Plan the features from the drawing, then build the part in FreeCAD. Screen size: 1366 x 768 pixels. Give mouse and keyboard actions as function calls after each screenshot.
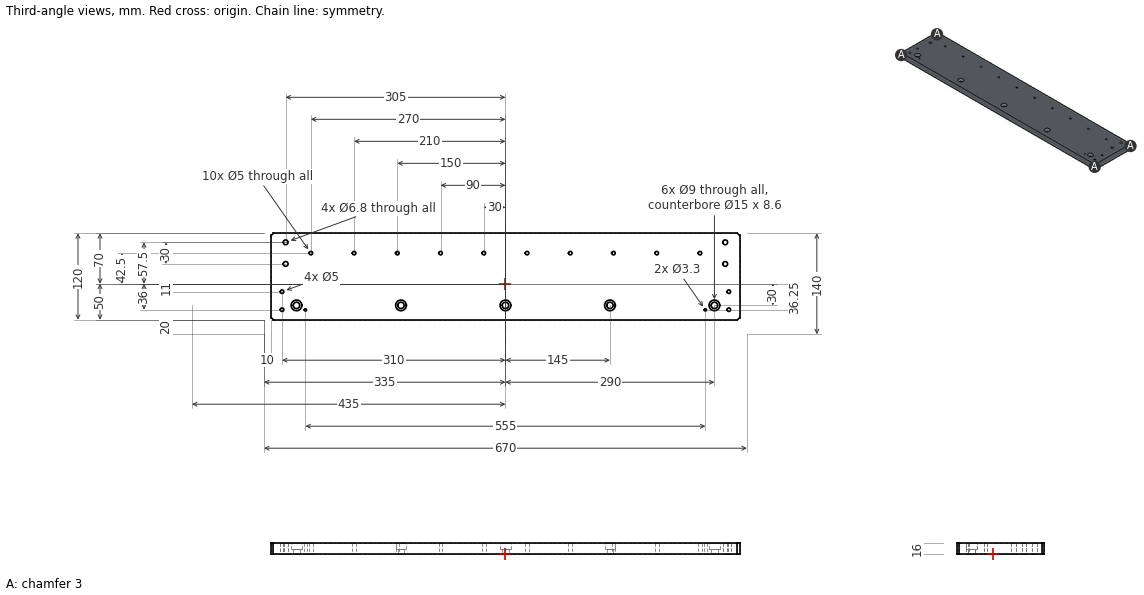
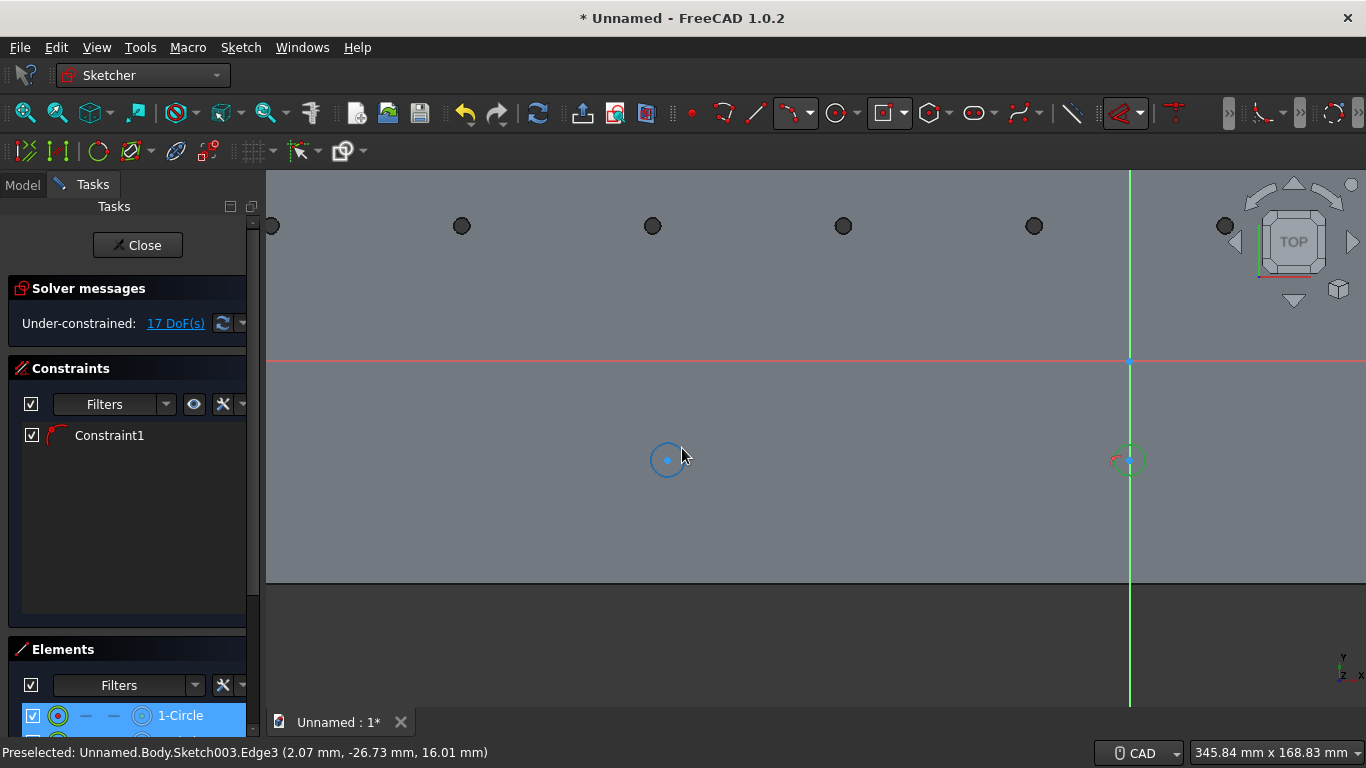
click(680, 448)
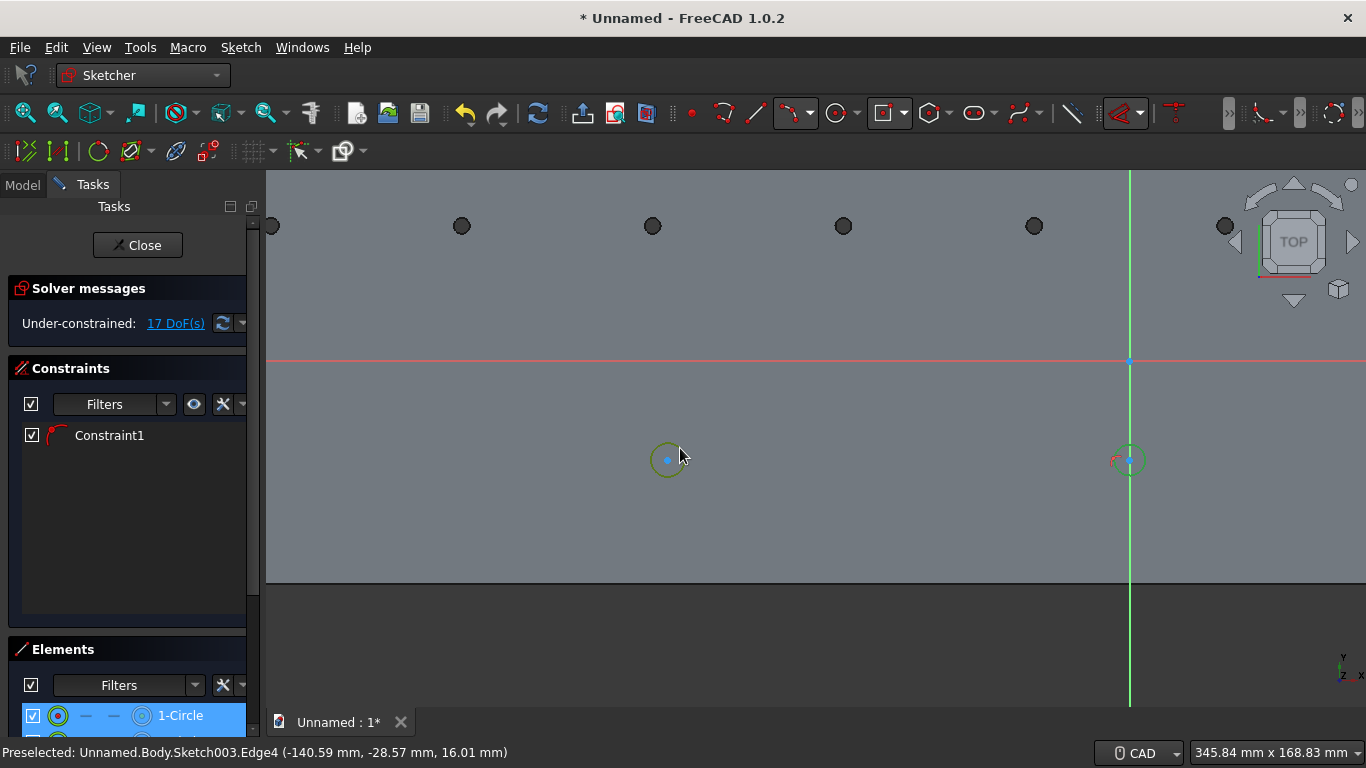
scroll(682, 448, down, 6)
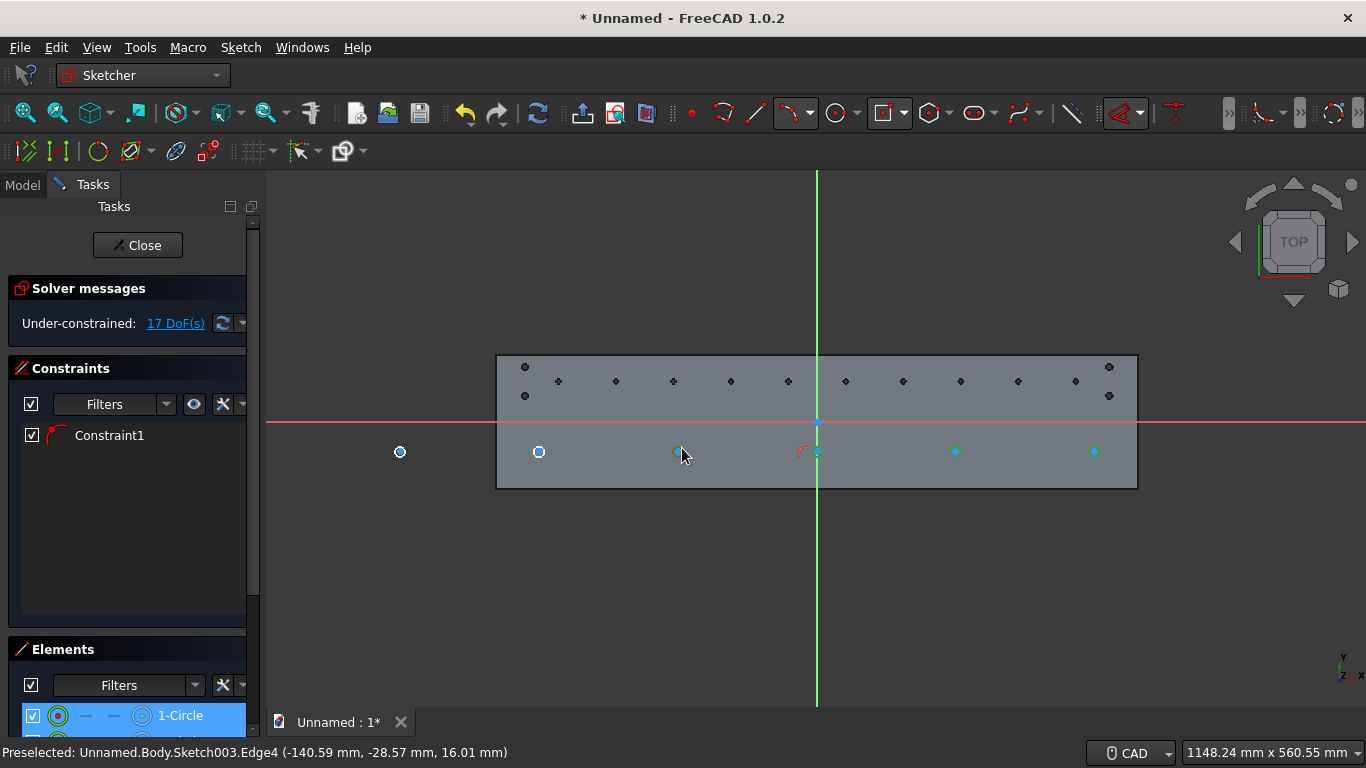
scroll(543, 448, up, 5)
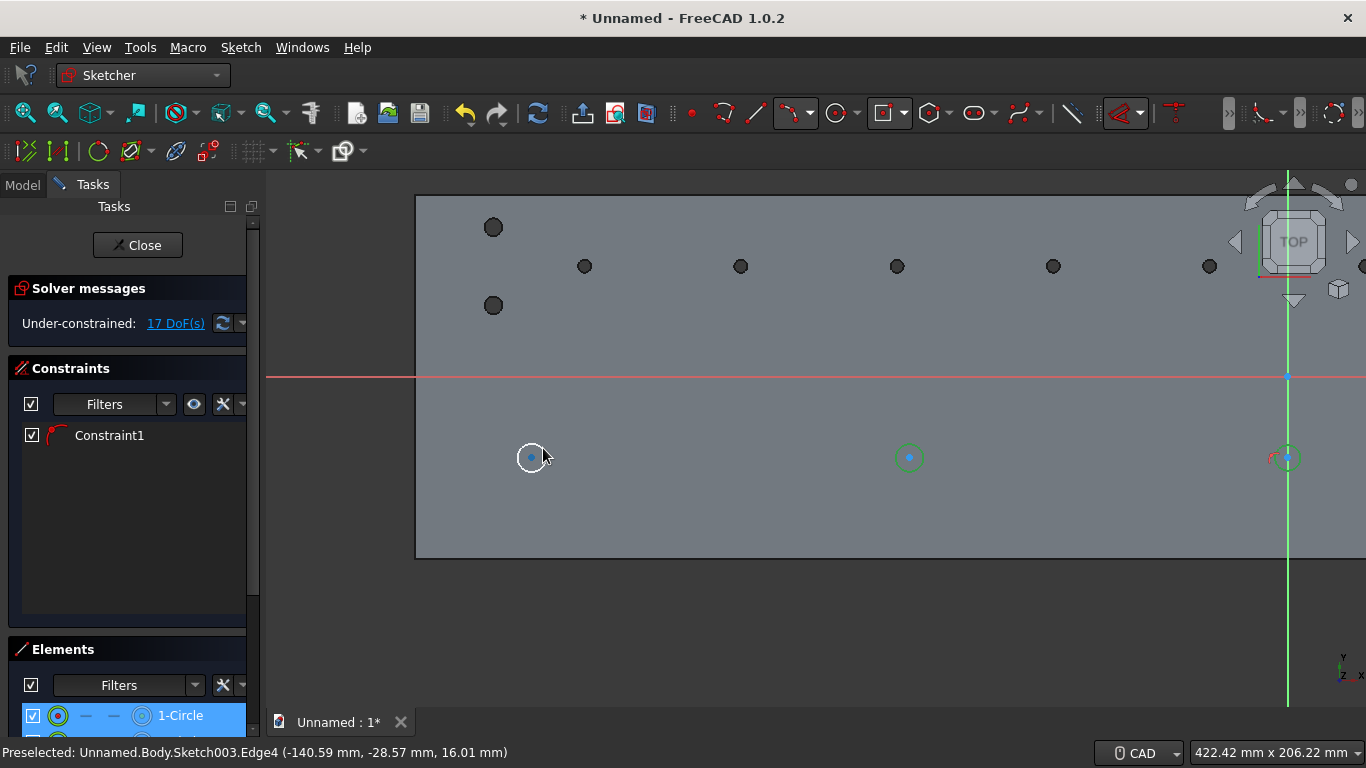
click(542, 448)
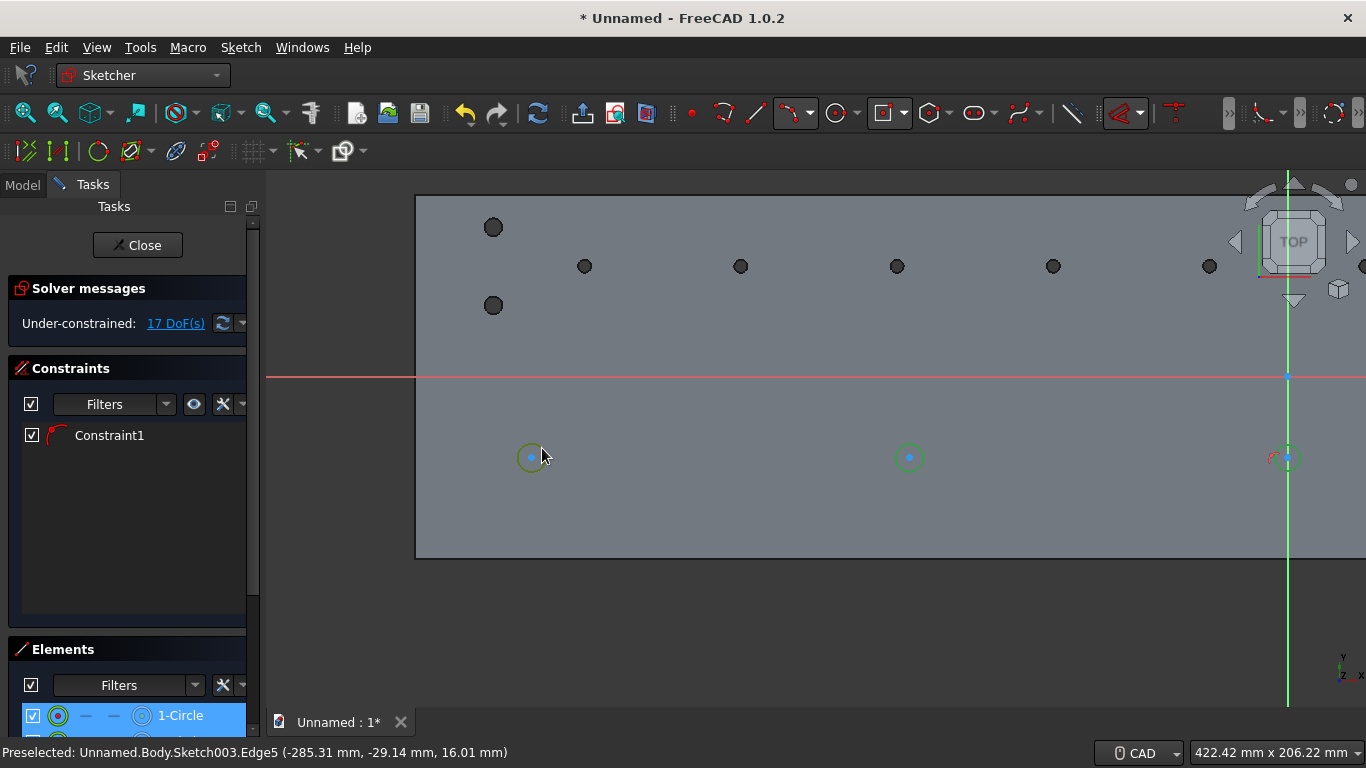
scroll(543, 448, down, 5)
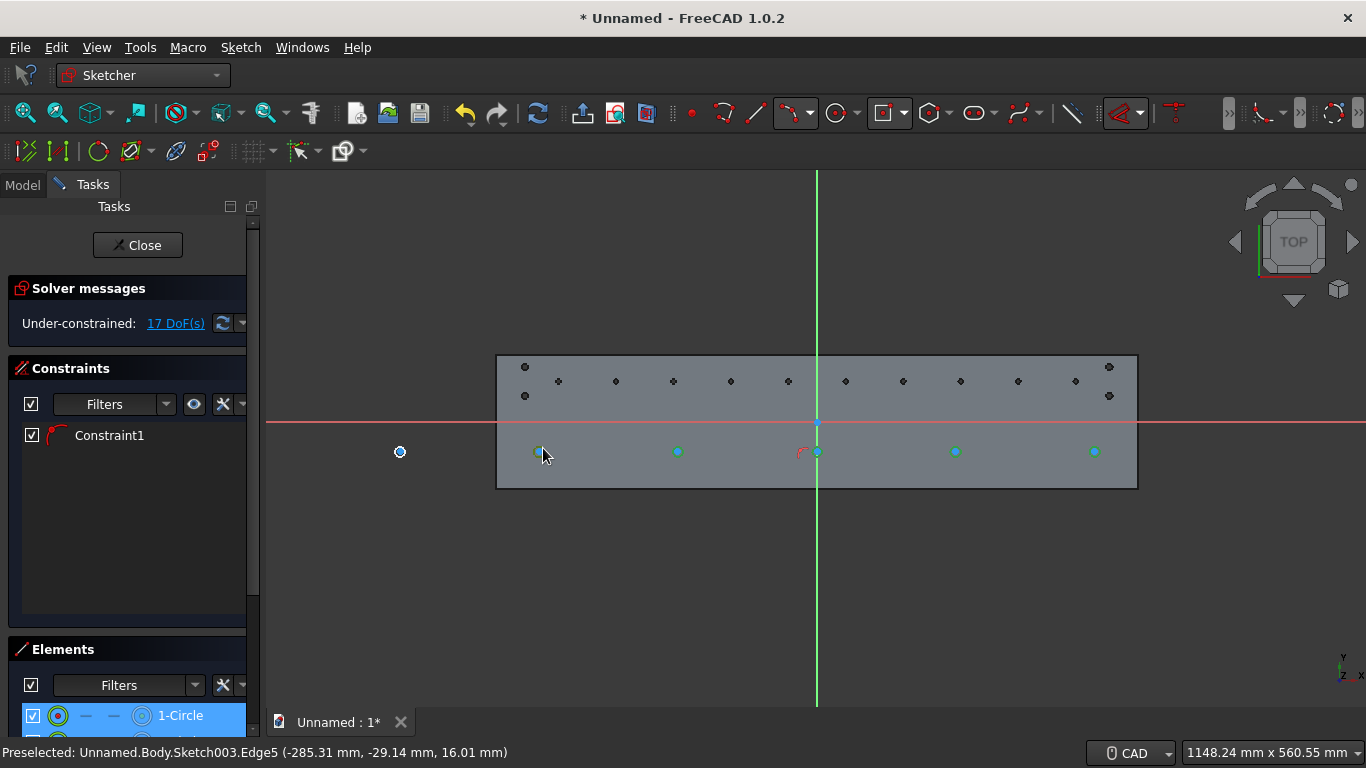
scroll(404, 448, up, 5)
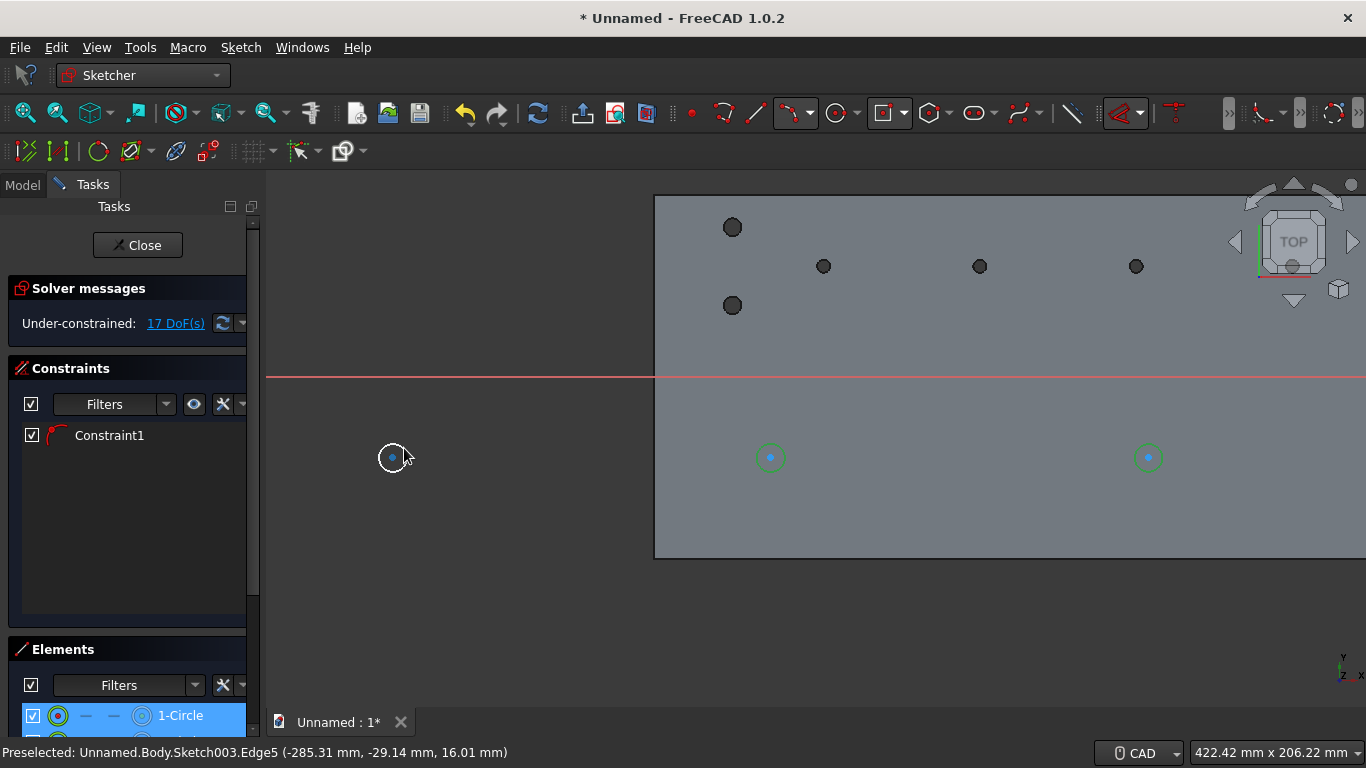
click(403, 448)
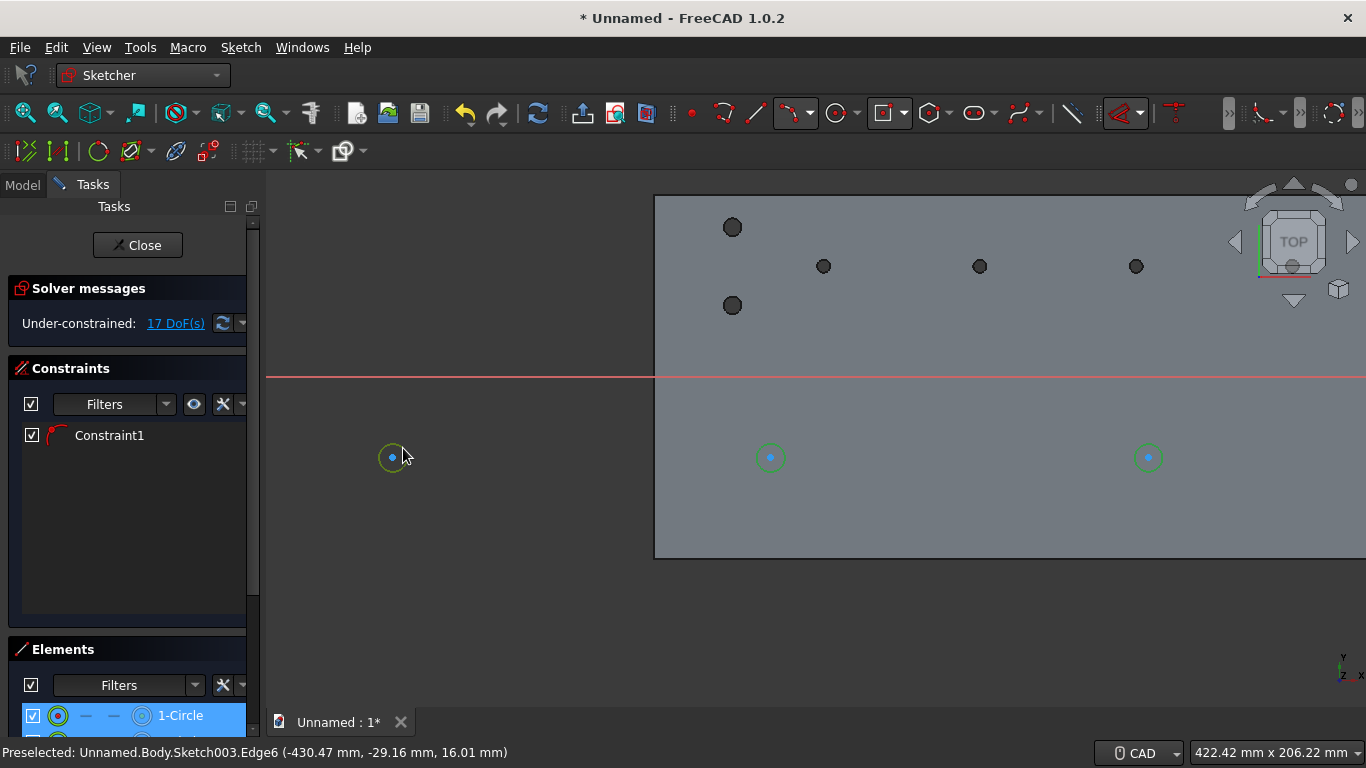
key(e)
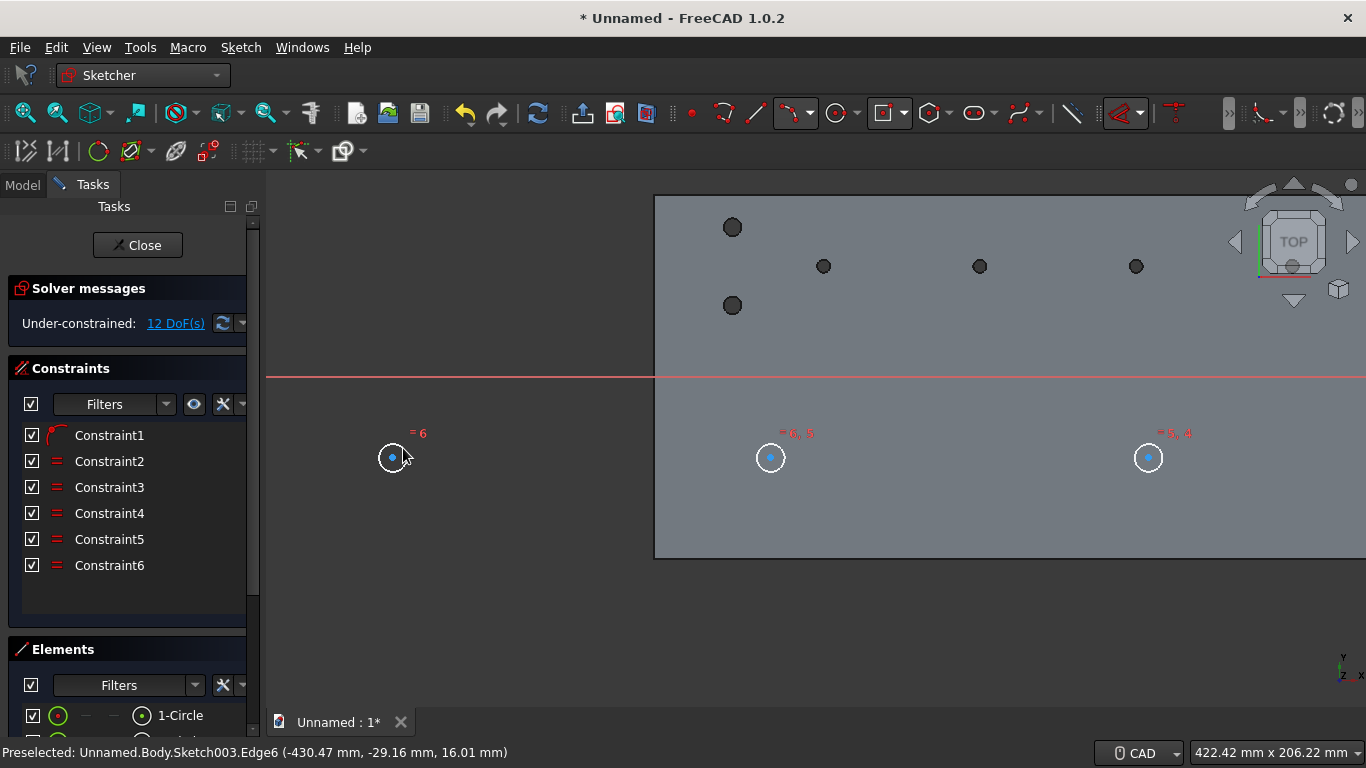
scroll(404, 448, down, 5)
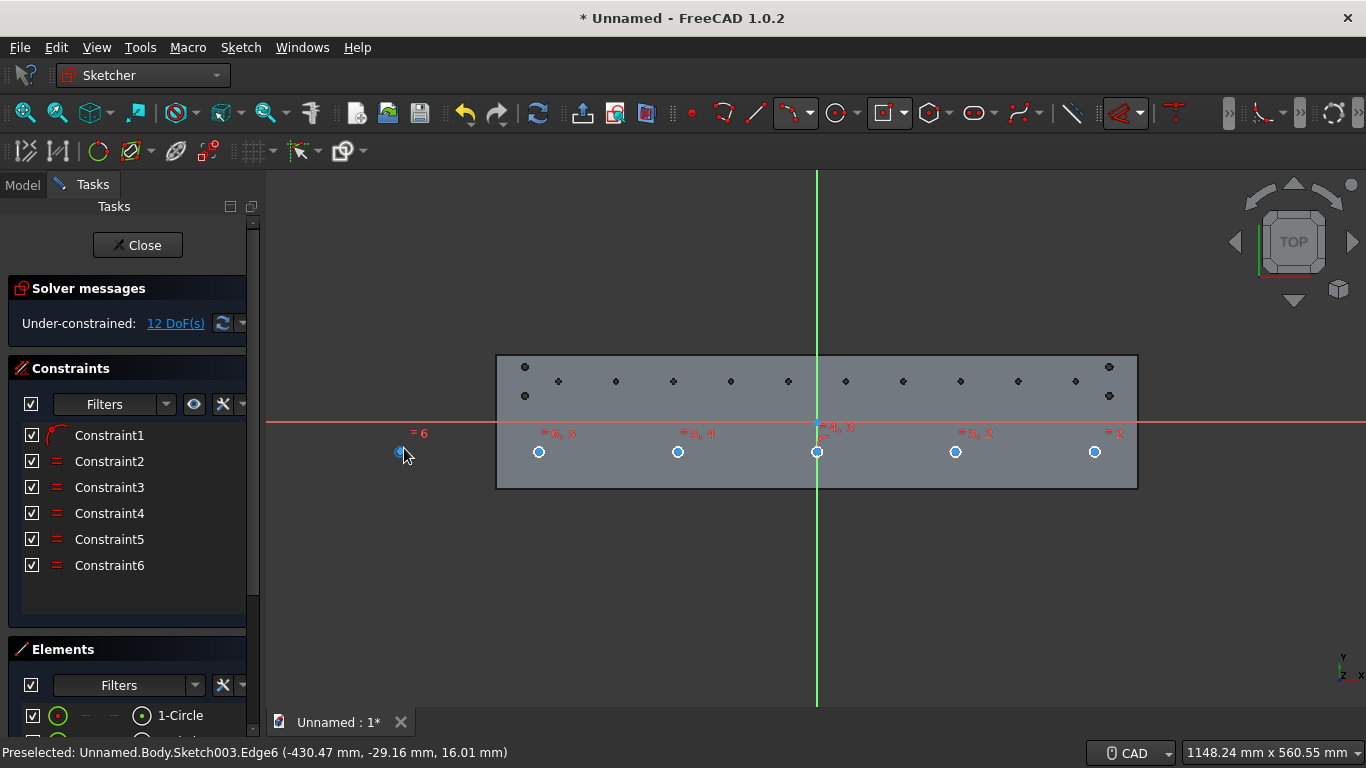
click(956, 452)